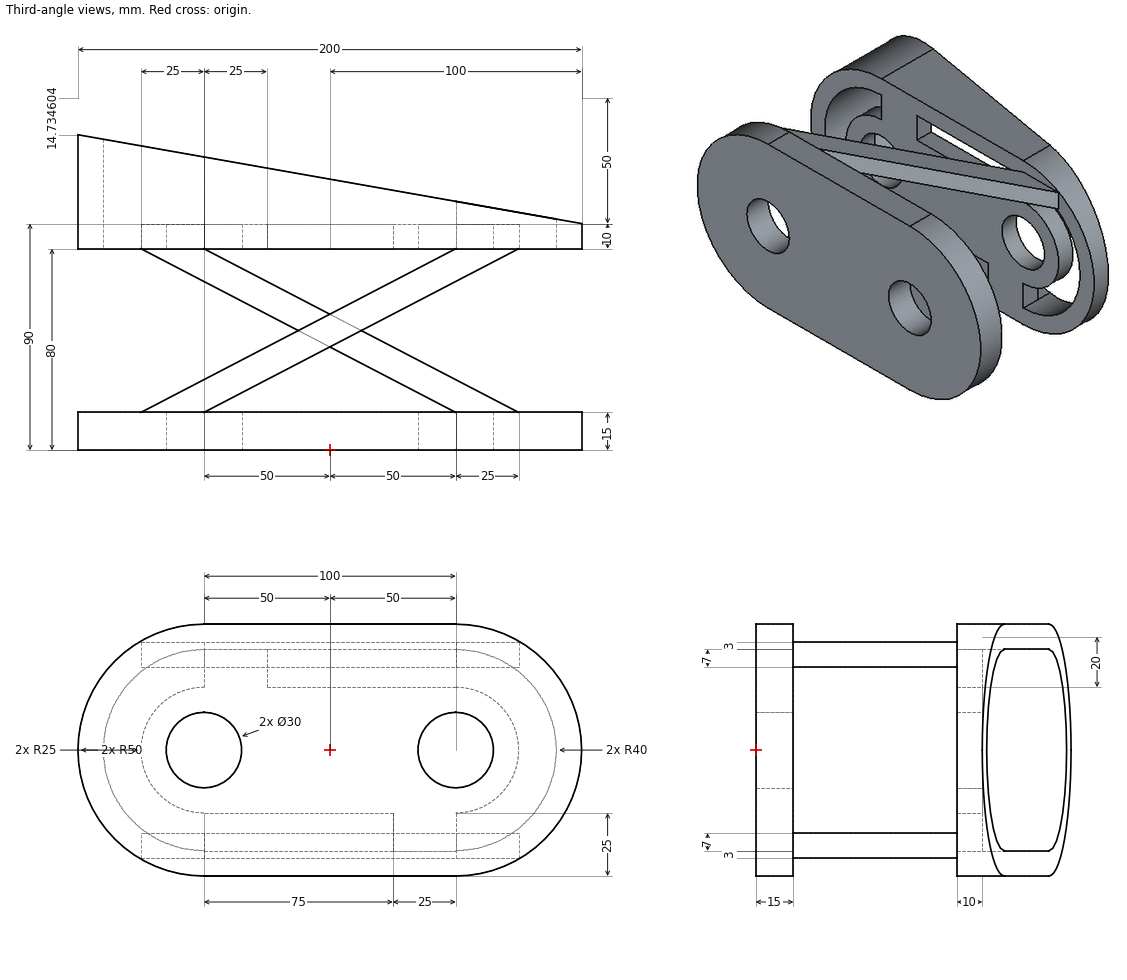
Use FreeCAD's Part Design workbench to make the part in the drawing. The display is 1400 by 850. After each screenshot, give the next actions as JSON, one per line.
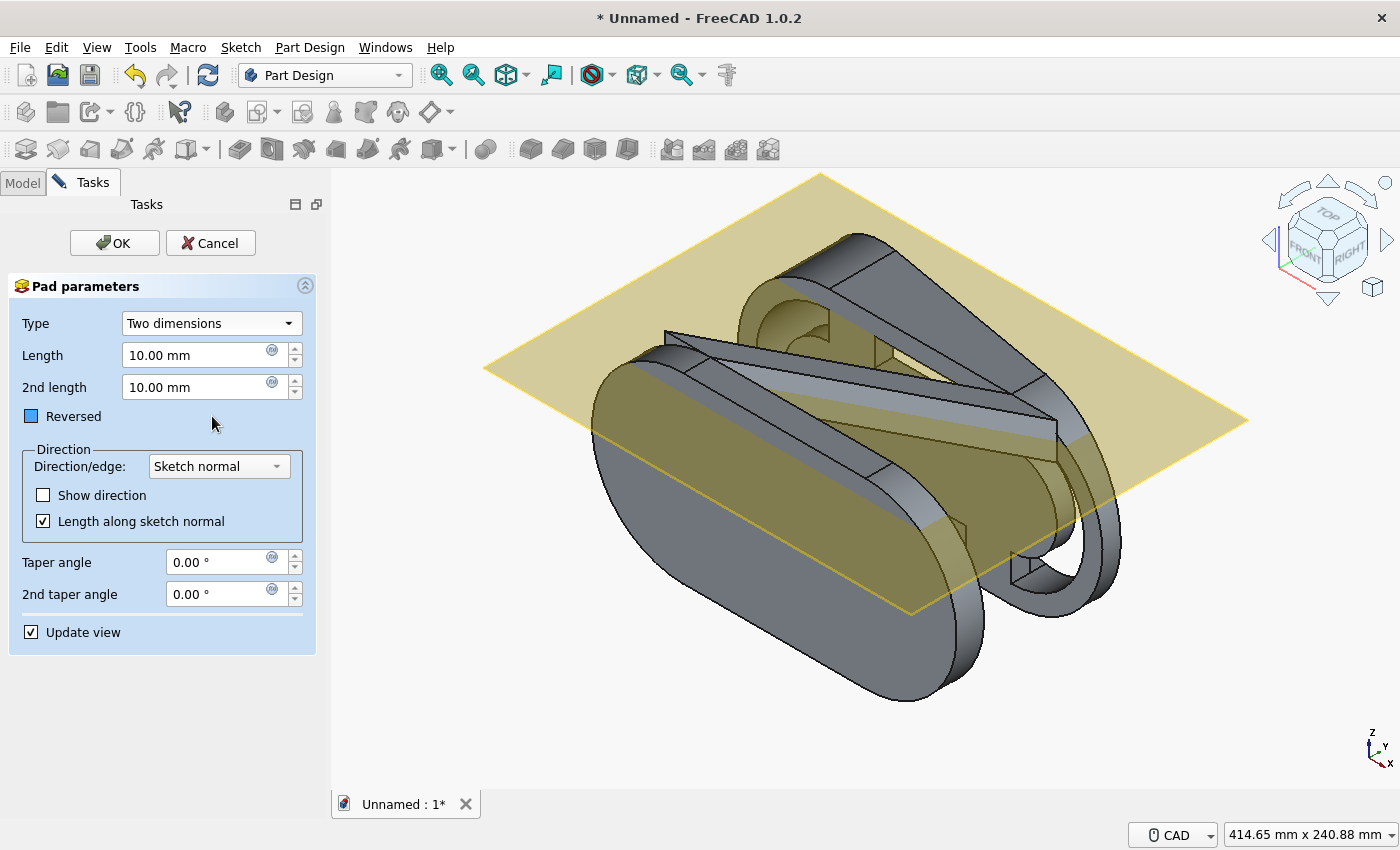
{"action": "triple_click", "coordinate": [204, 355]}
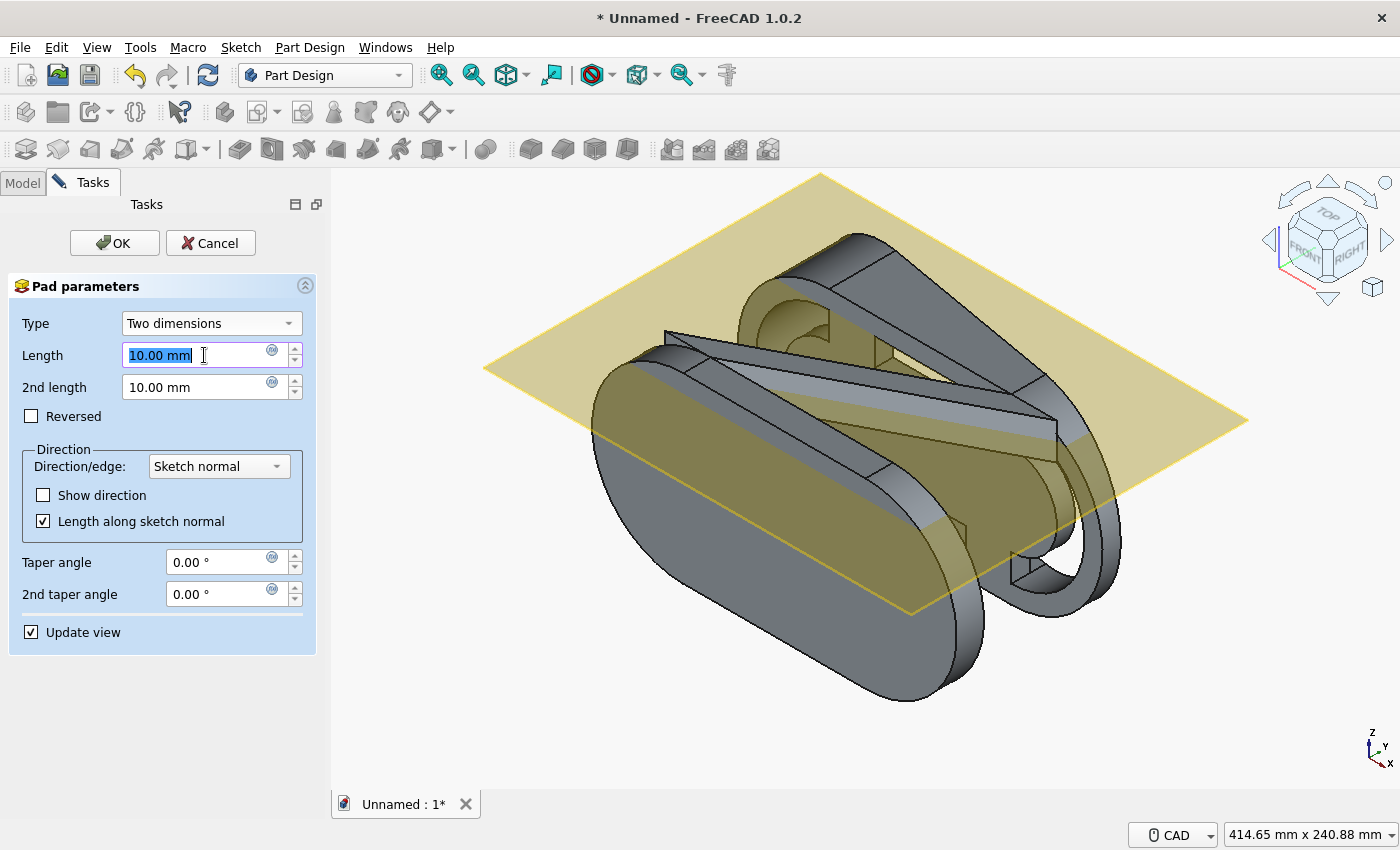
{"action": "type", "text": "7"}
{"action": "key", "text": "Tab"}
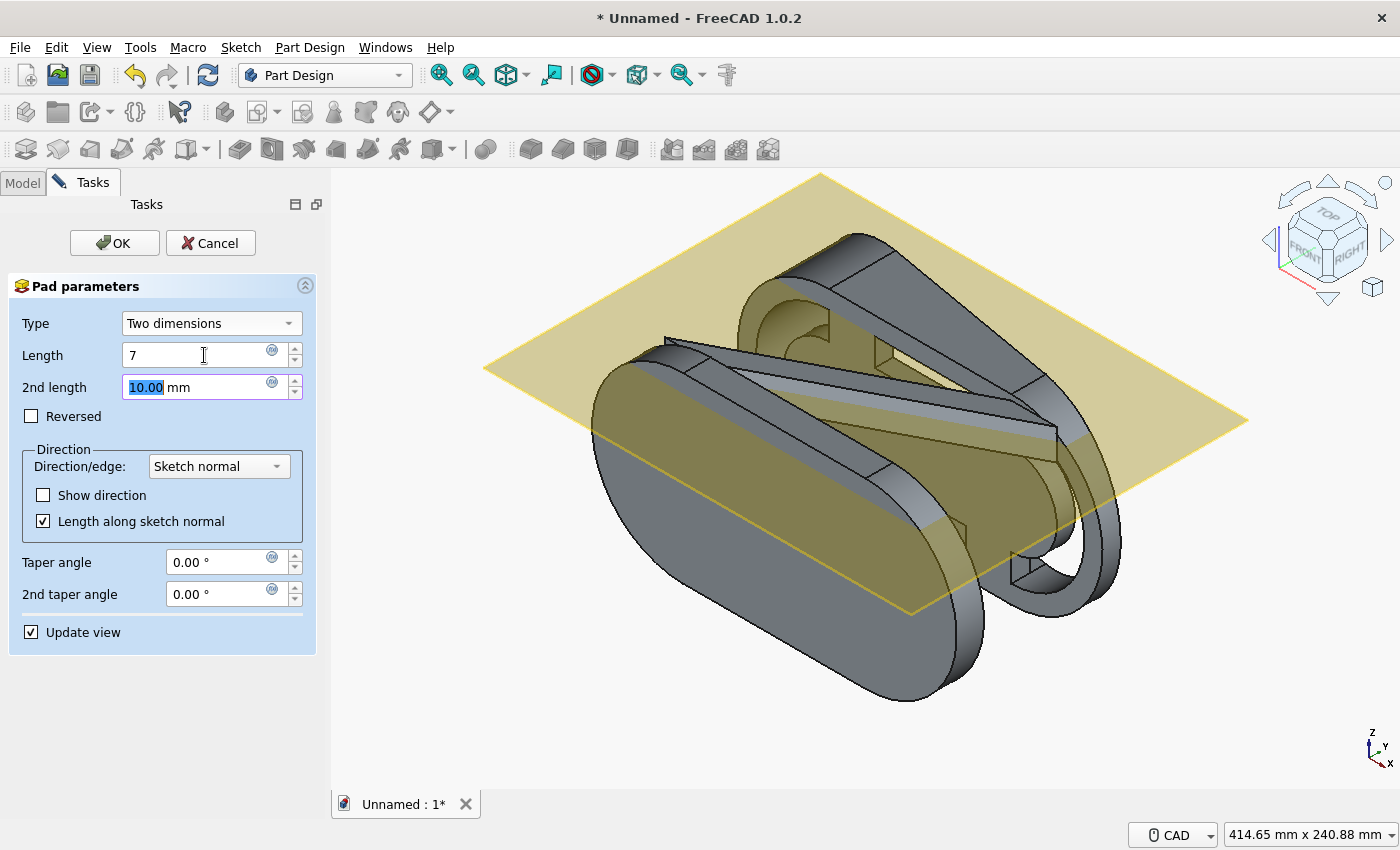
{"action": "type", "text": "3"}
{"action": "key", "text": "Tab"}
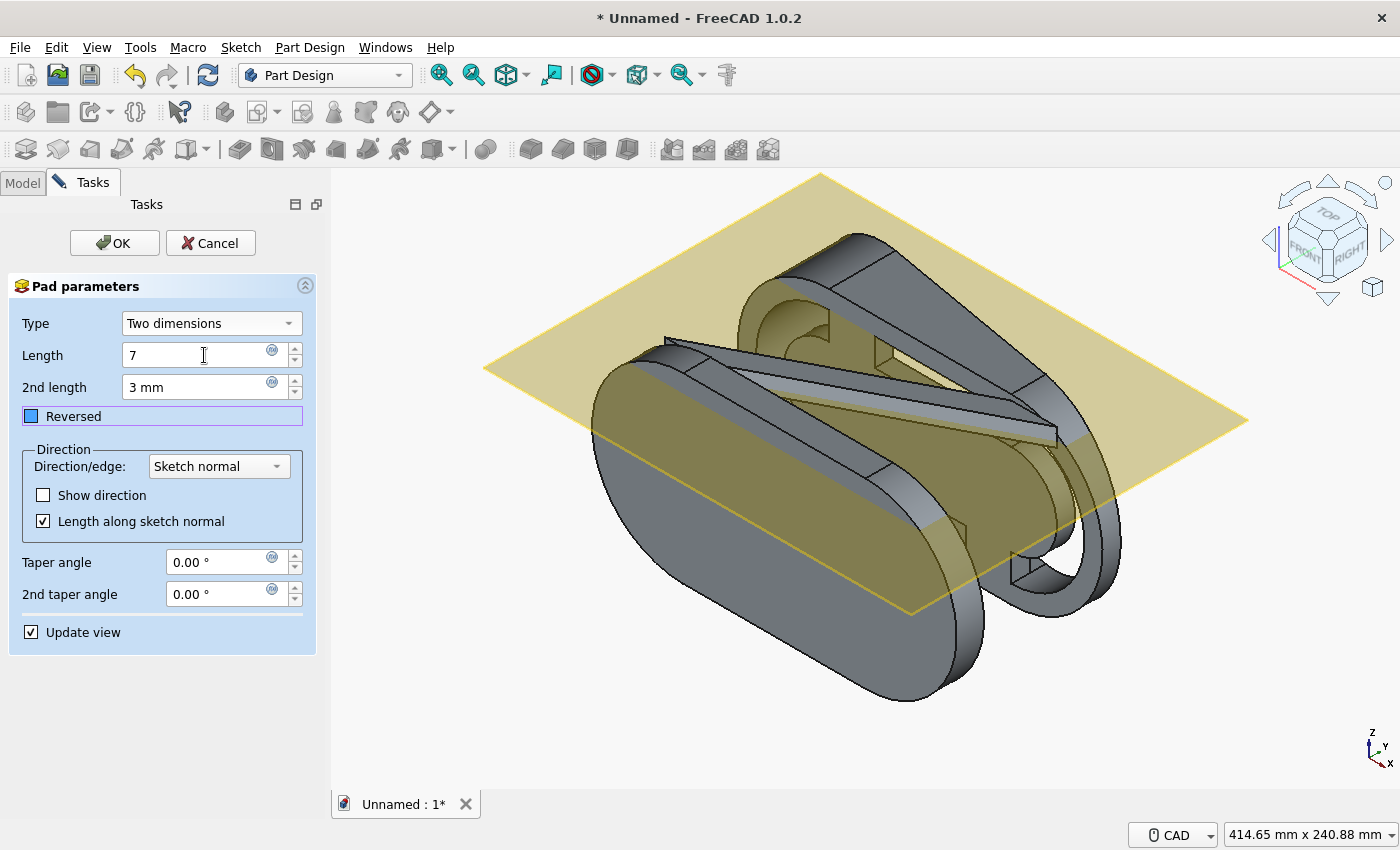
{"action": "left_click", "coordinate": [30, 416]}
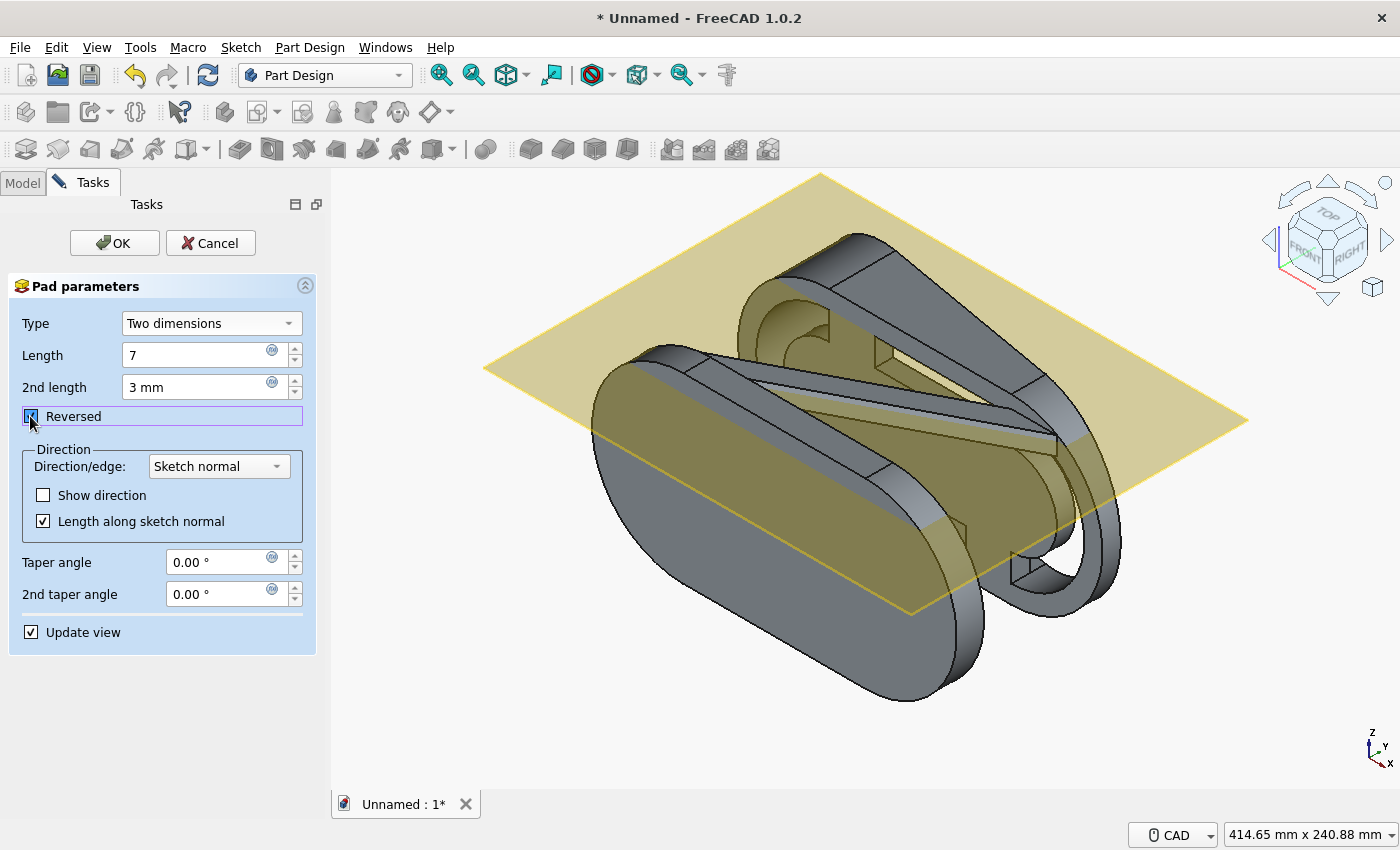
{"action": "left_click", "coordinate": [115, 243]}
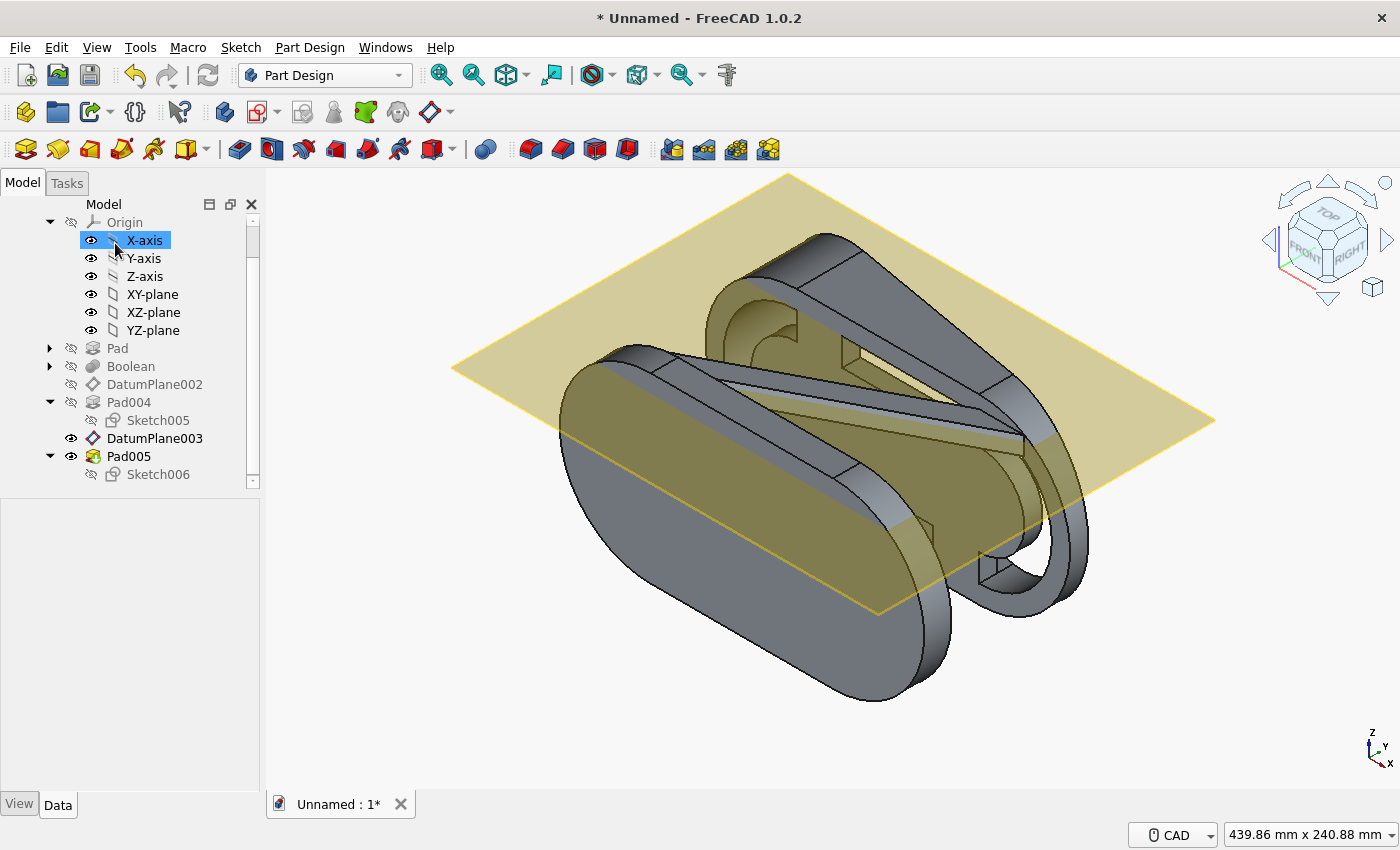
{"action": "left_click", "coordinate": [116, 438]}
{"action": "key", "text": "space"}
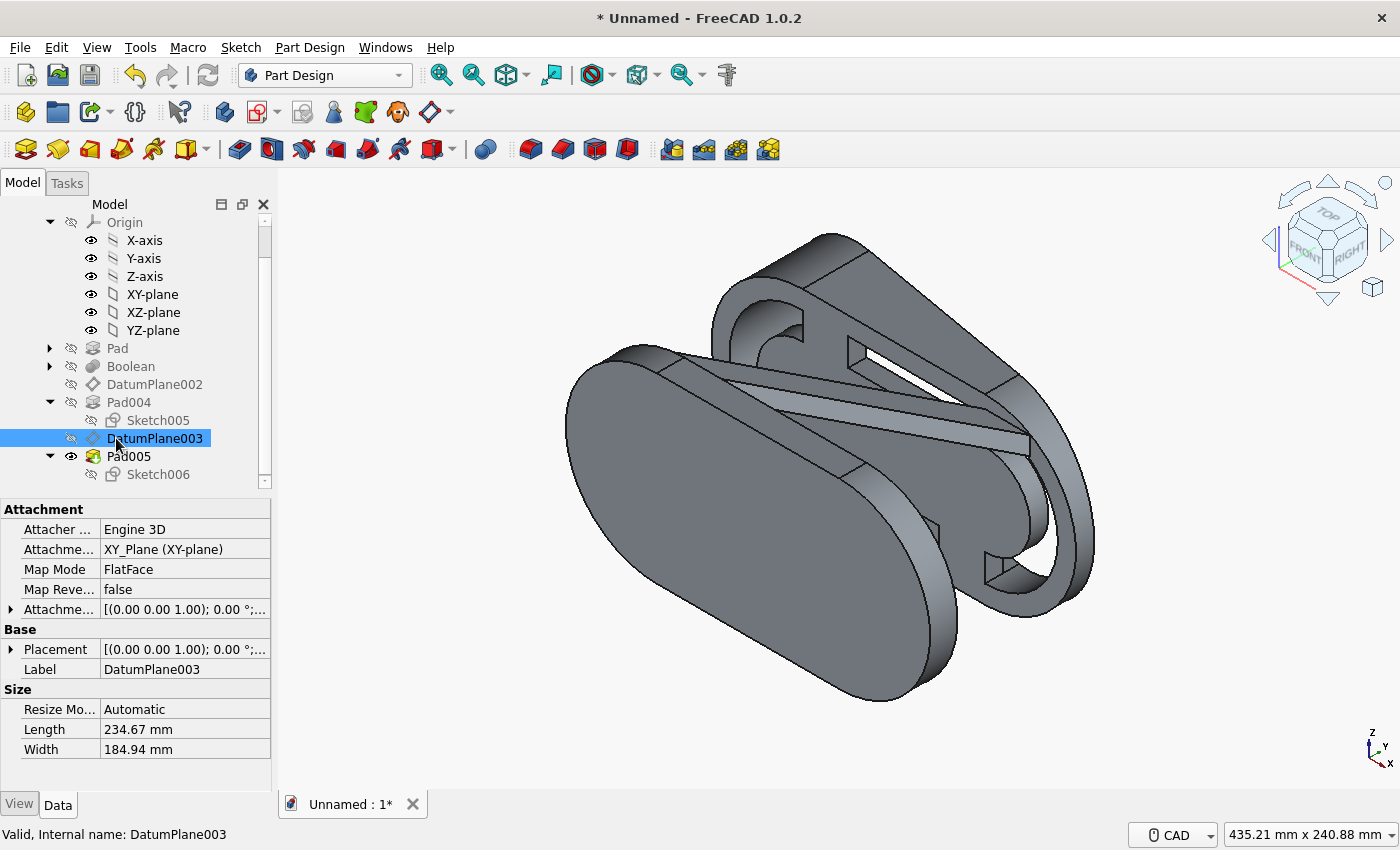
{"action": "left_click", "coordinate": [136, 312]}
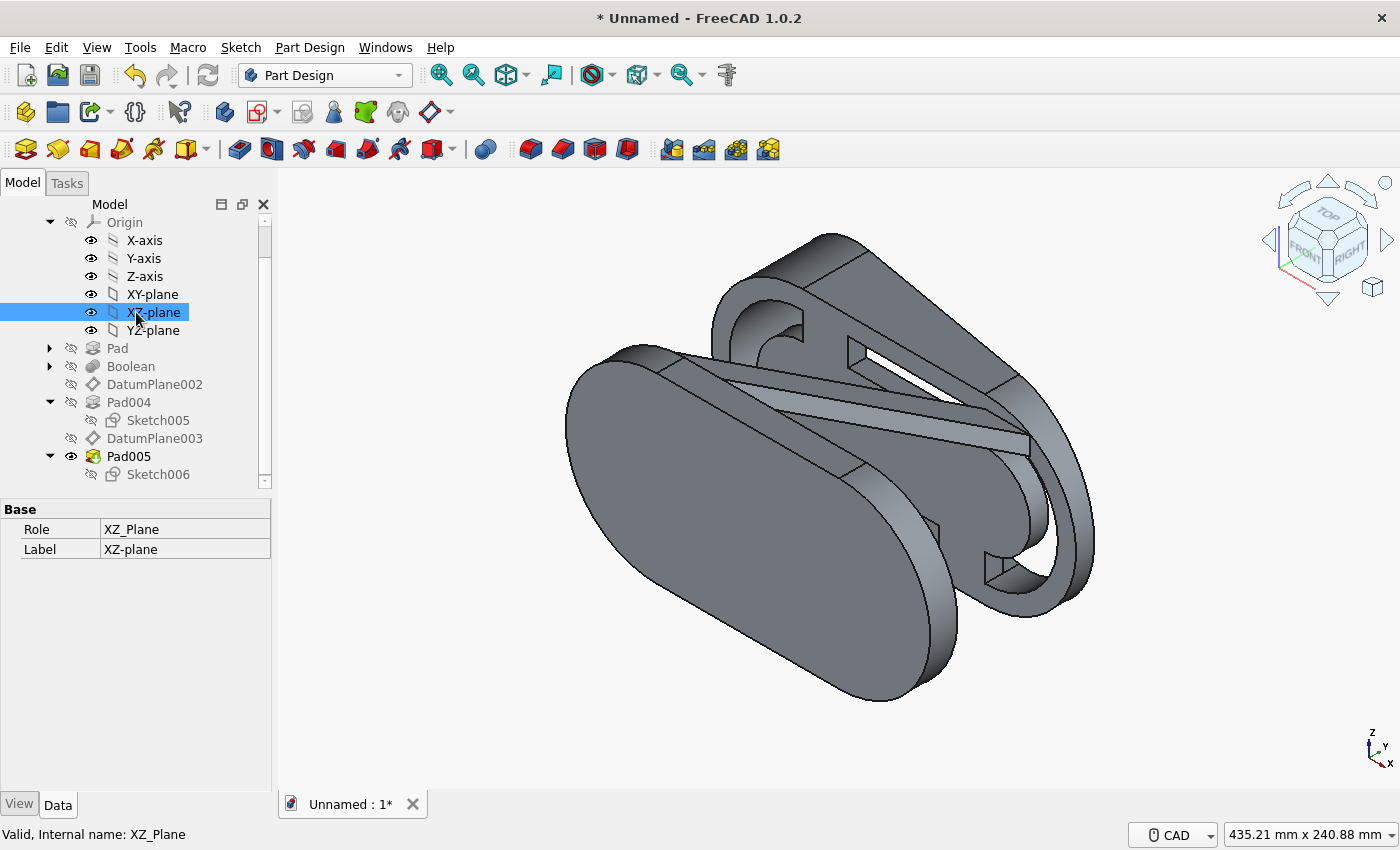
{"action": "left_click", "coordinate": [430, 112]}